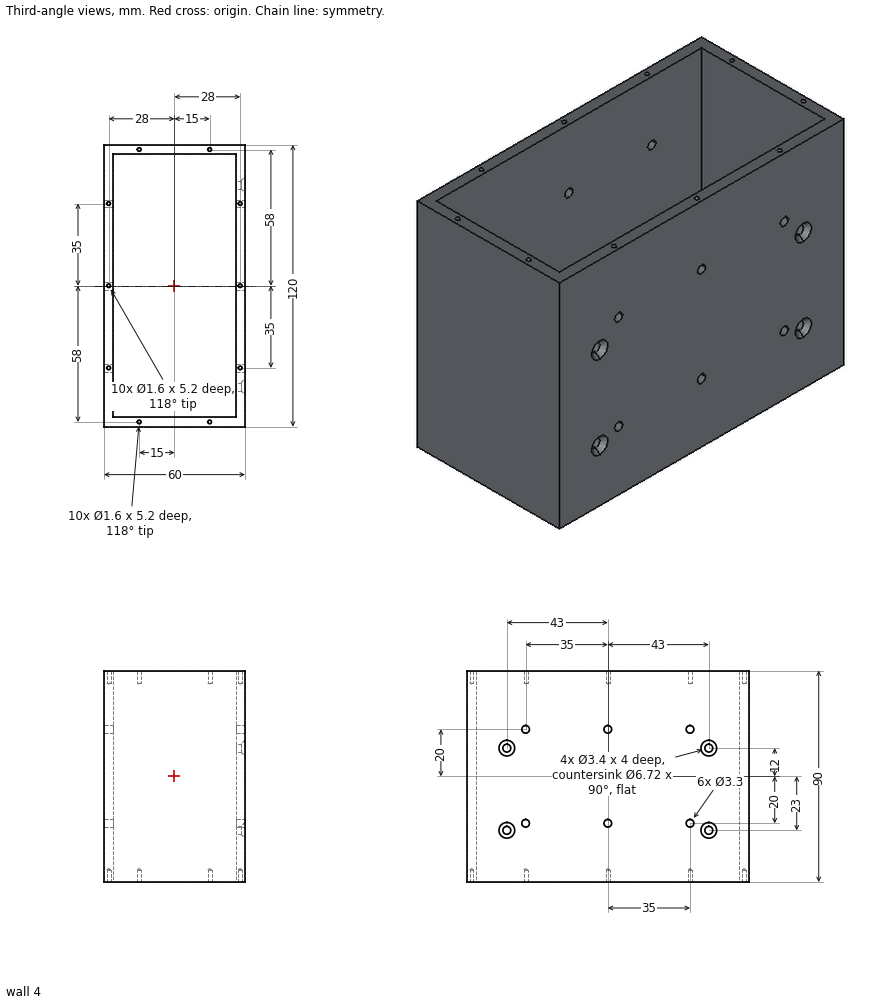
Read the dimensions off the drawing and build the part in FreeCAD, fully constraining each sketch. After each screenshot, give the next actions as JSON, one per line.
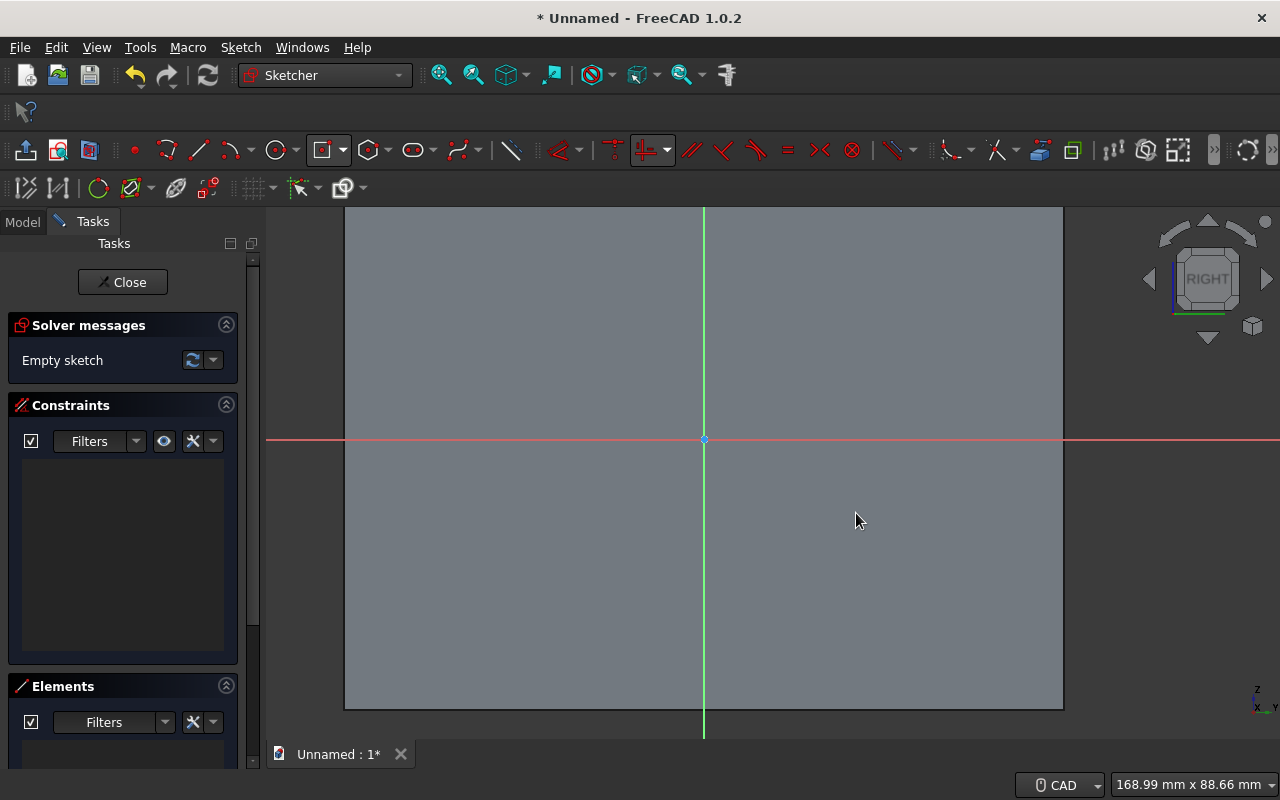
{"action": "left_click", "coordinate": [276, 150]}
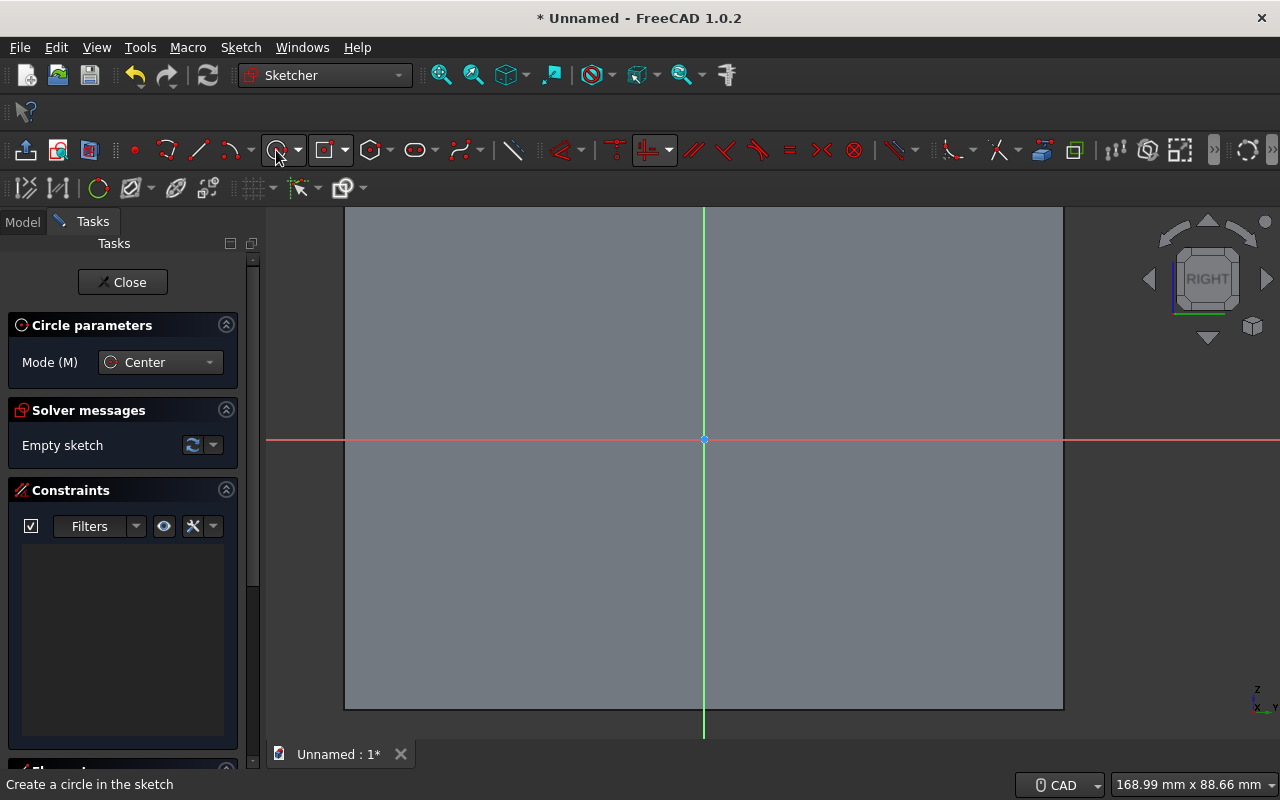
{"action": "scroll", "coordinate": [962, 368], "scroll_direction": "up", "scroll_amount": 4}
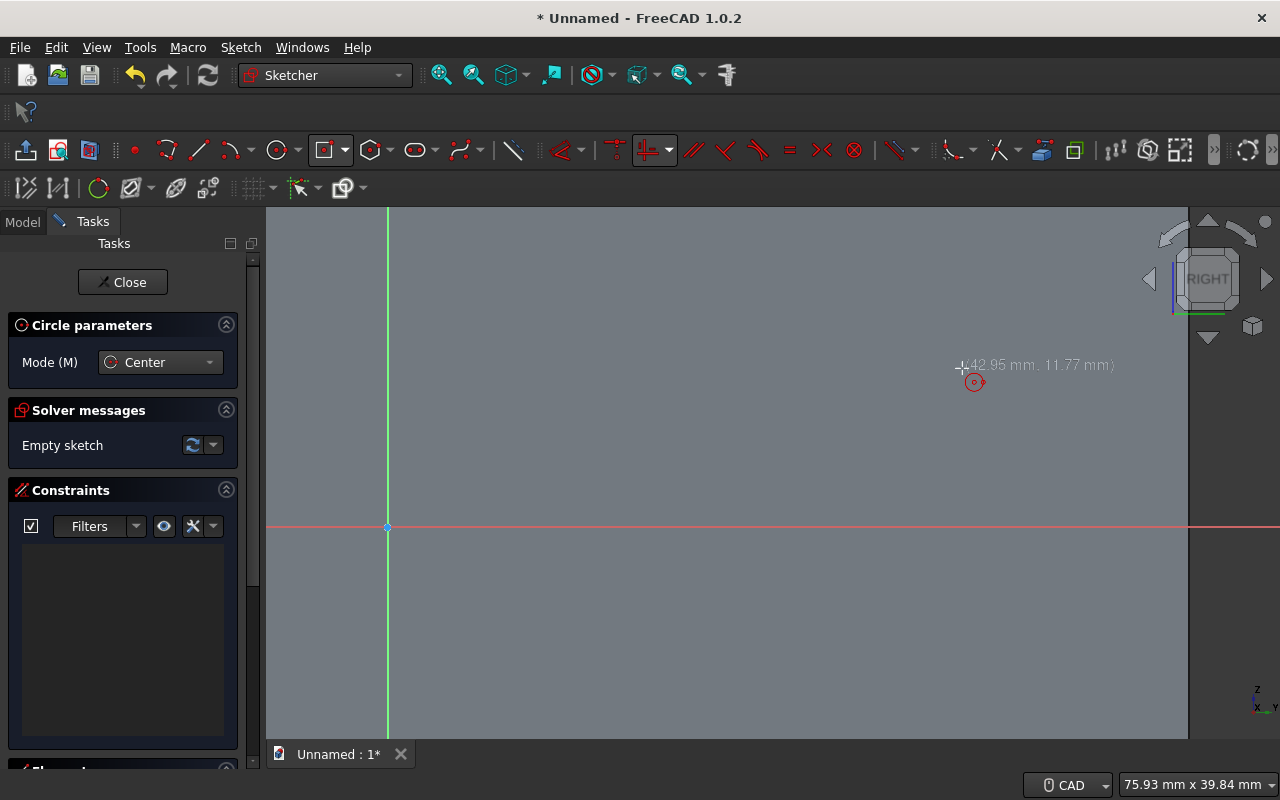
{"action": "left_click", "coordinate": [962, 367]}
{"action": "mouse_move", "coordinate": [978, 351]}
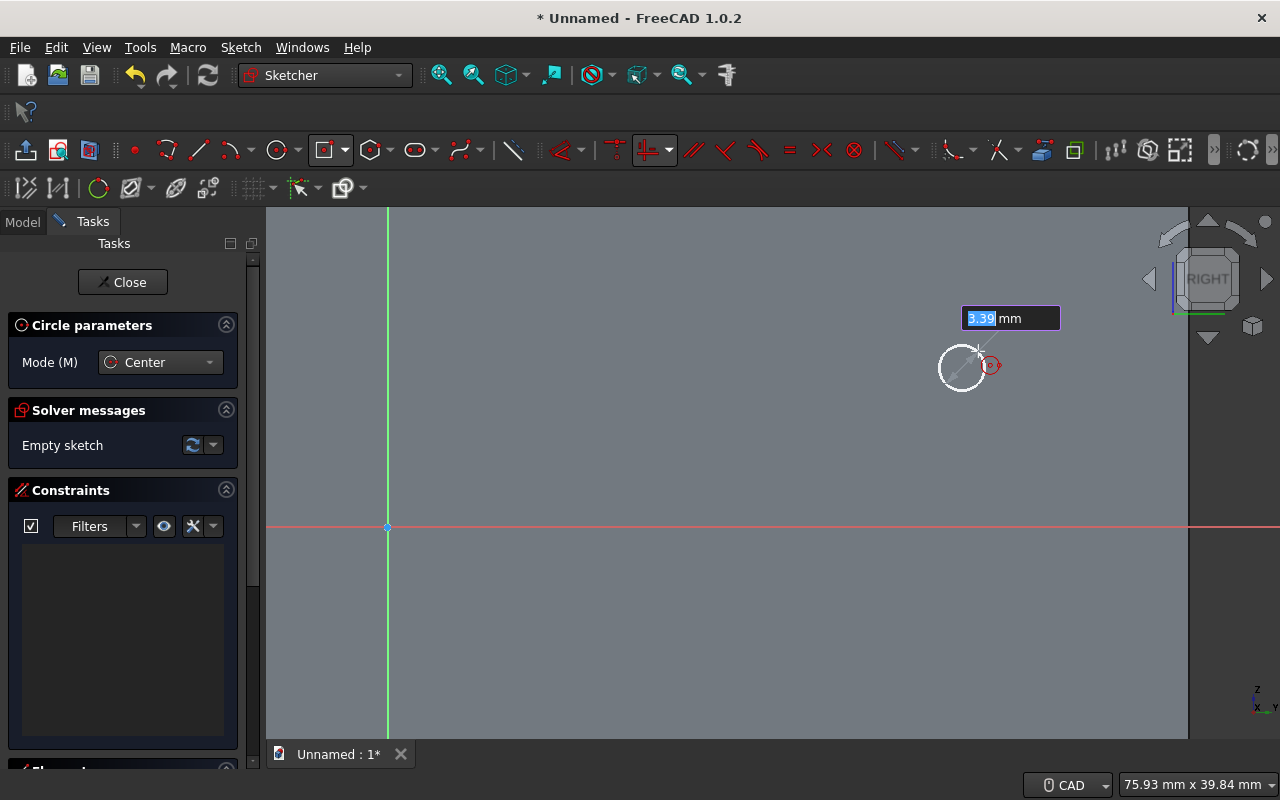
{"action": "type", "text": "3.4"}
{"action": "key", "text": "Return"}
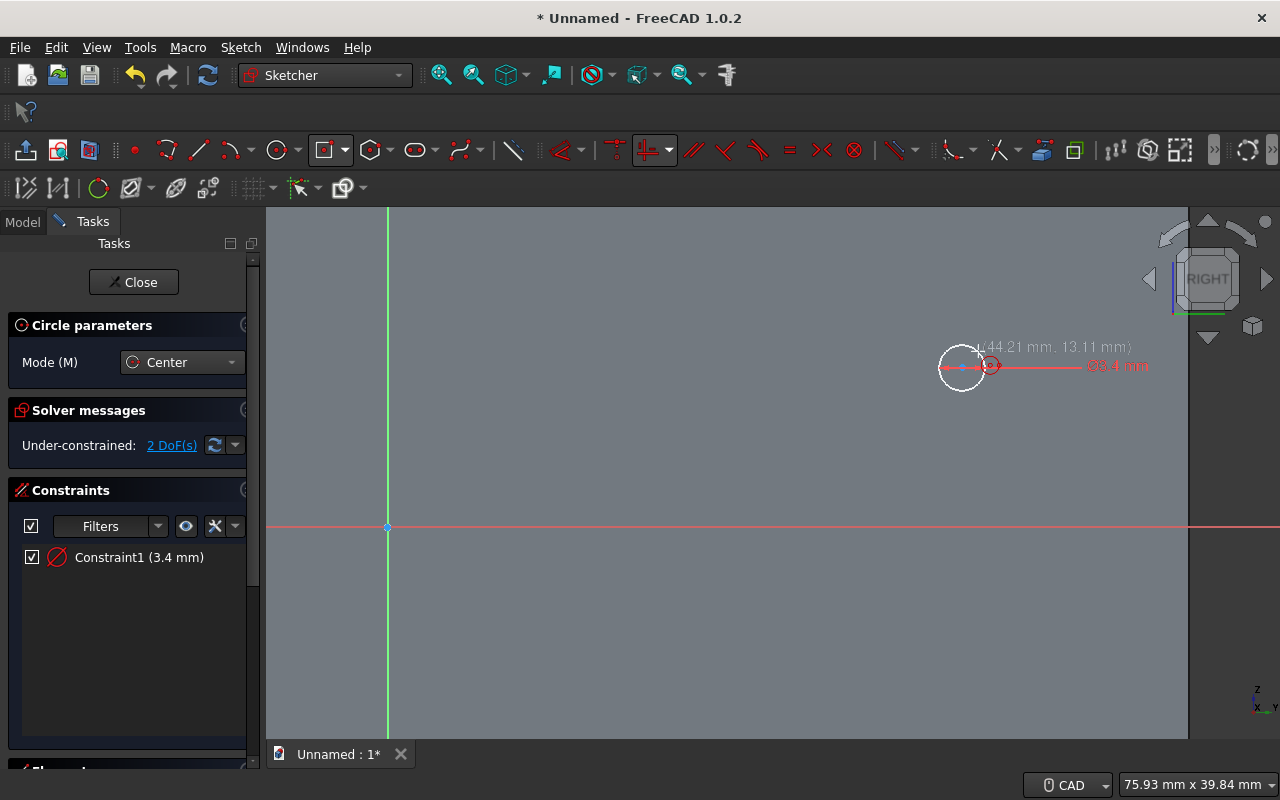
{"action": "scroll", "coordinate": [963, 369], "scroll_direction": "down", "scroll_amount": 4}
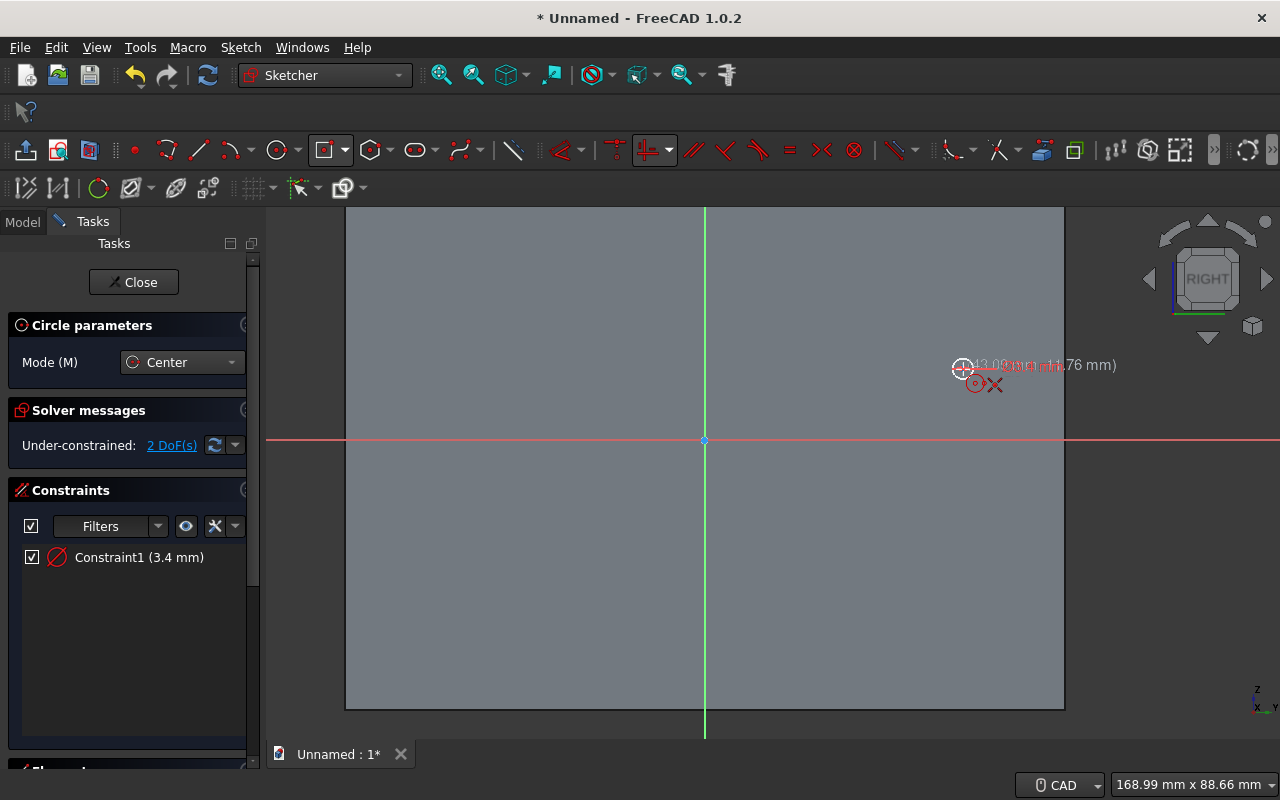
{"action": "scroll", "coordinate": [963, 578], "scroll_direction": "up", "scroll_amount": 4}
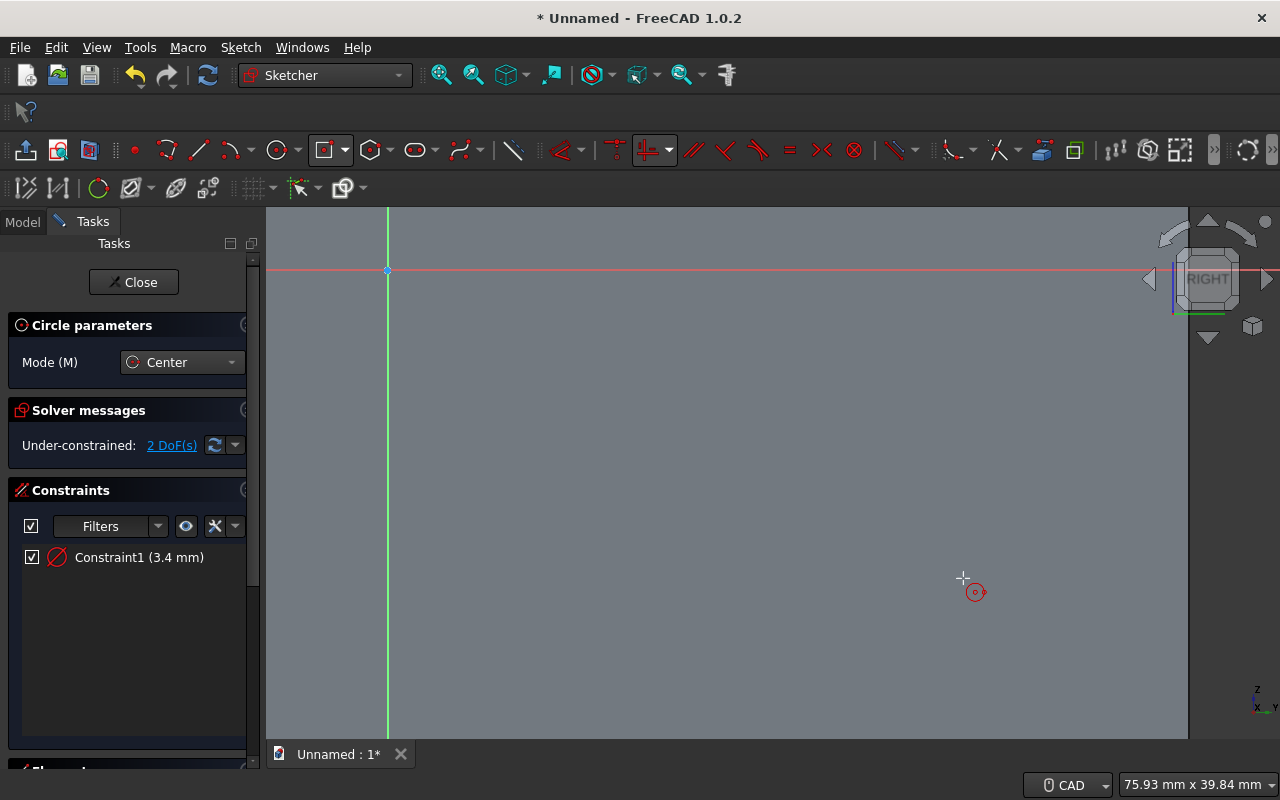
{"action": "left_click", "coordinate": [962, 578]}
{"action": "mouse_move", "coordinate": [978, 562]}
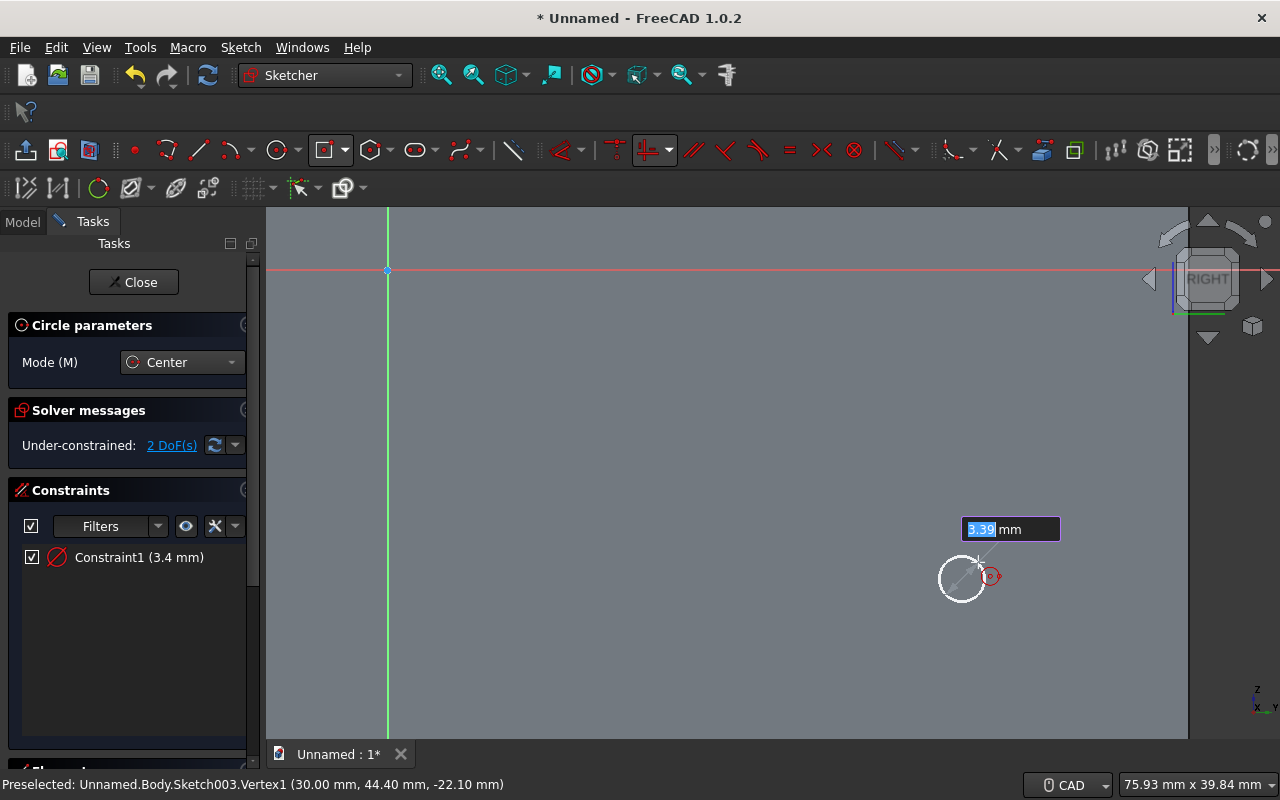
{"action": "type", "text": "3.4"}
{"action": "key", "text": "Return"}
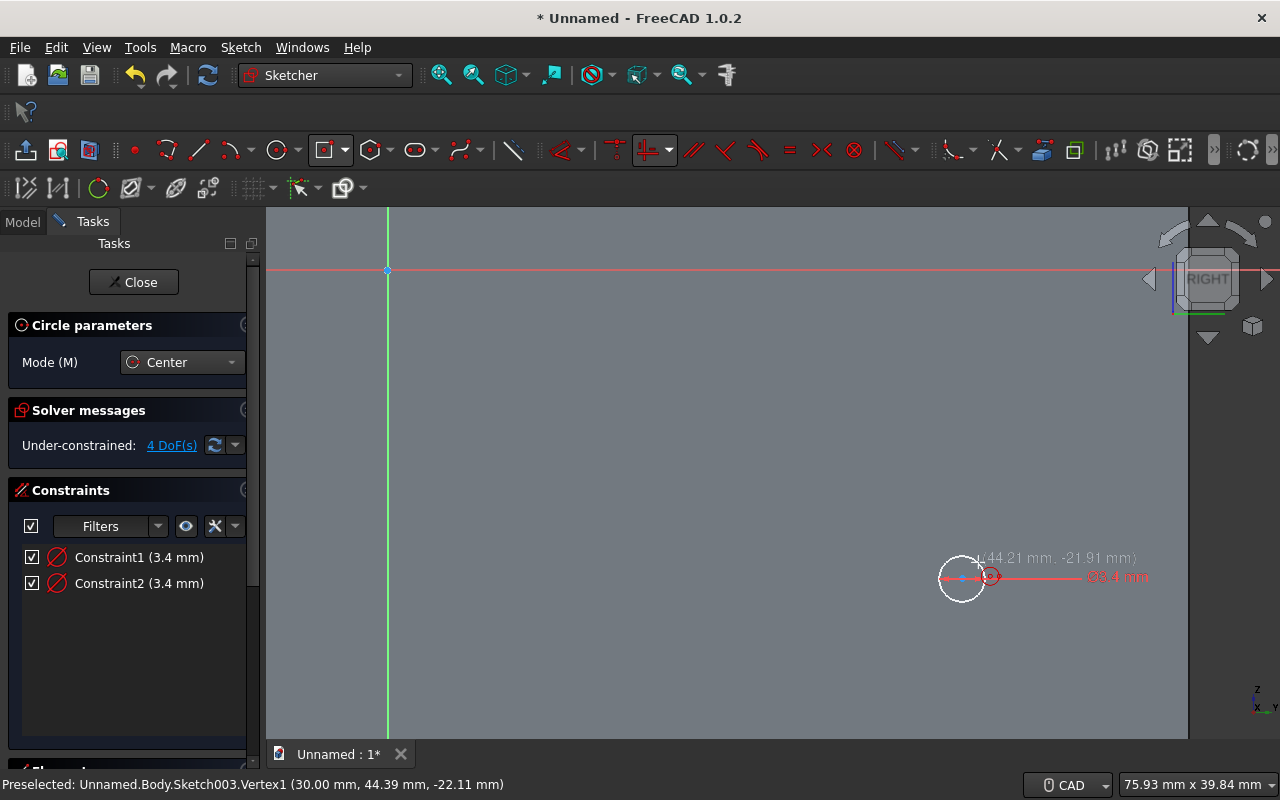
{"action": "scroll", "coordinate": [963, 578], "scroll_direction": "down", "scroll_amount": 4}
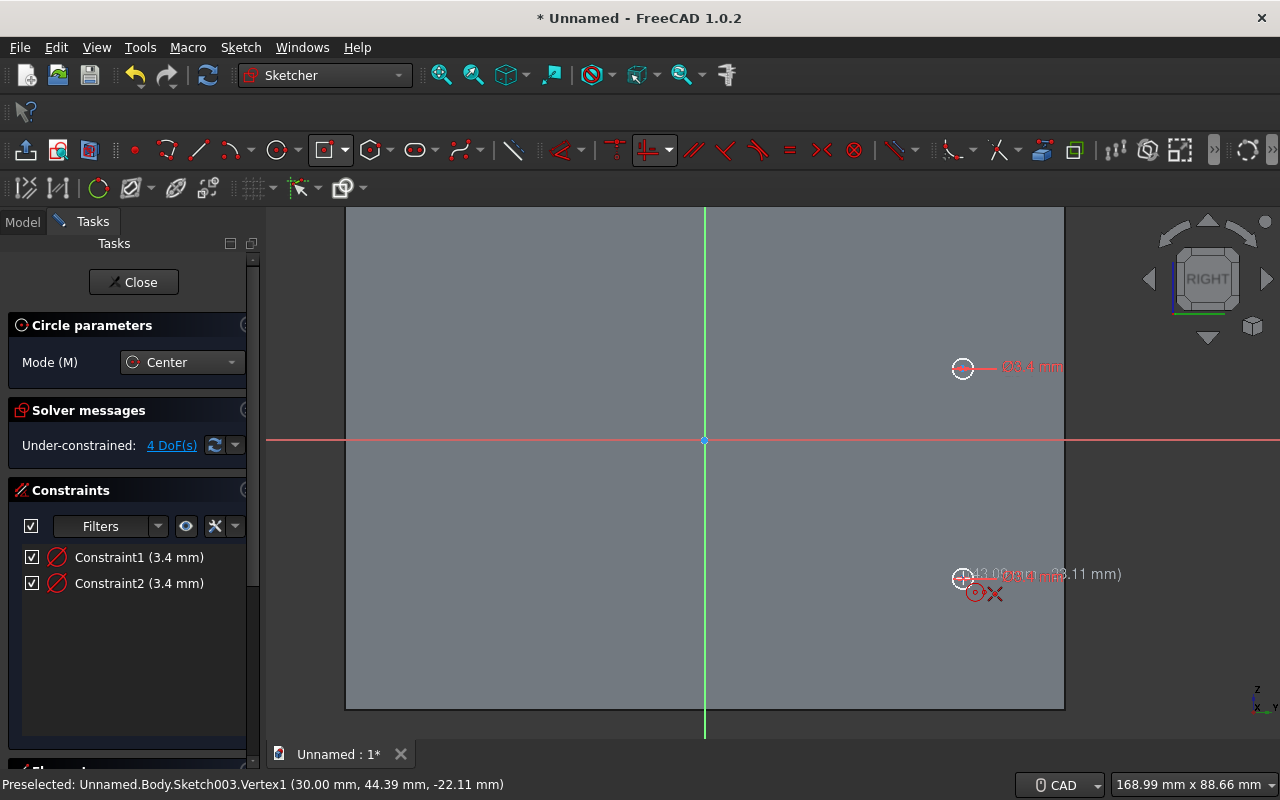
{"action": "scroll", "coordinate": [447, 368], "scroll_direction": "up", "scroll_amount": 4}